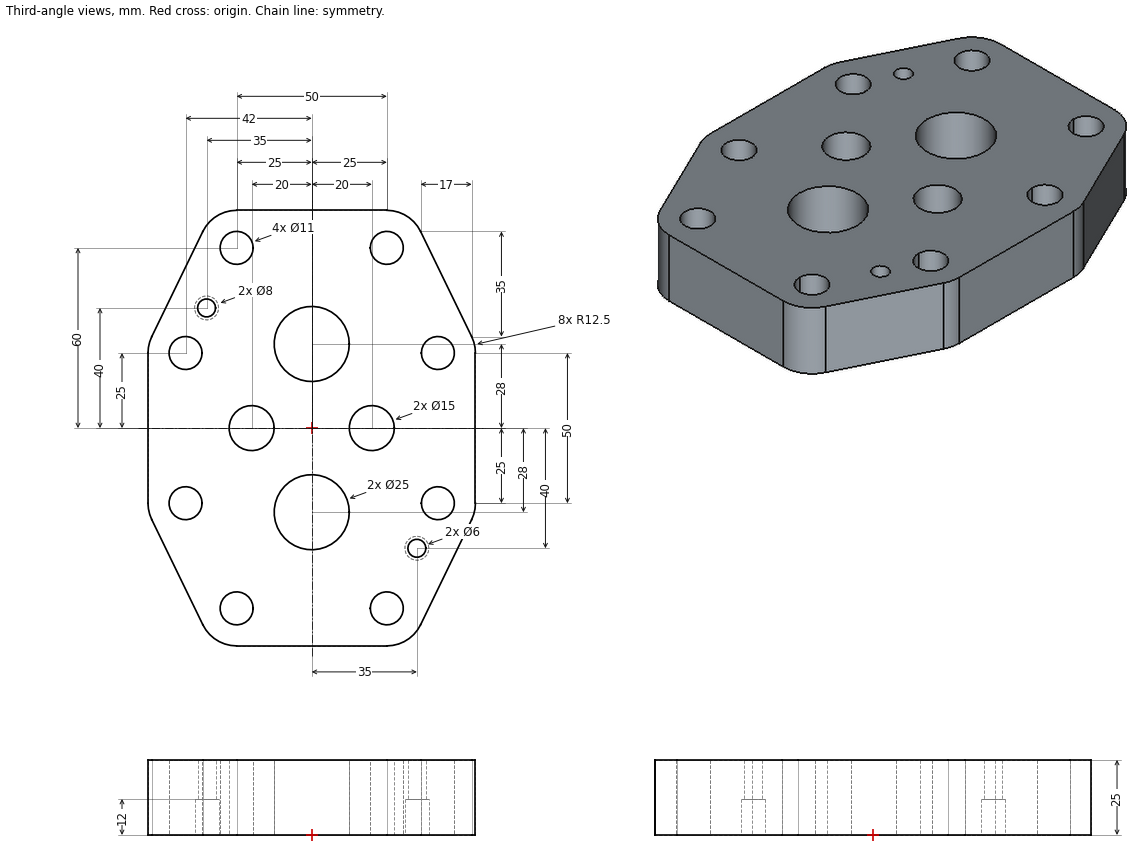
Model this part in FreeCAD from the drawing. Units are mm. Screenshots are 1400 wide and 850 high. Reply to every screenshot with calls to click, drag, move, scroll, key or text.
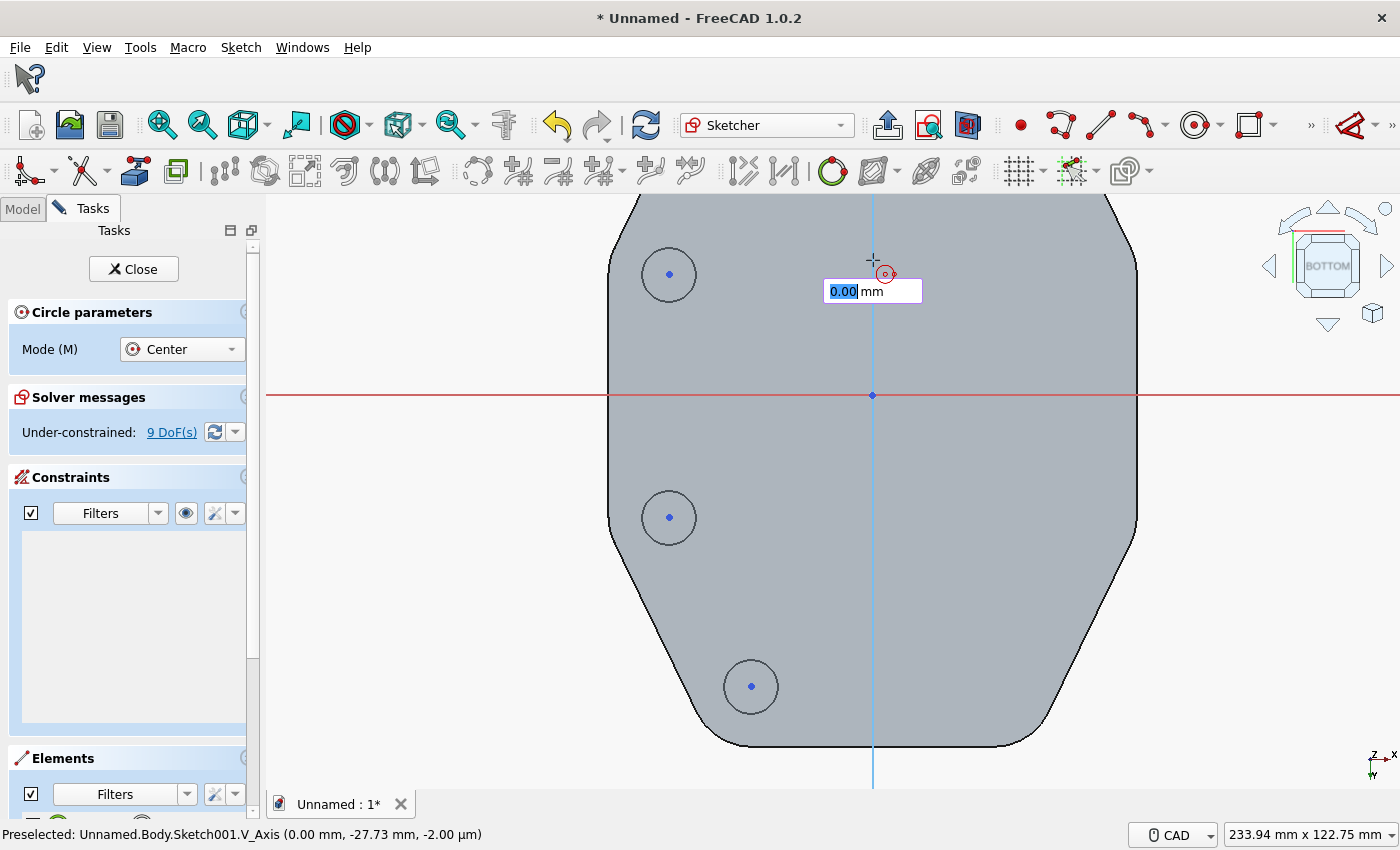
scroll(692, 608, down, 3)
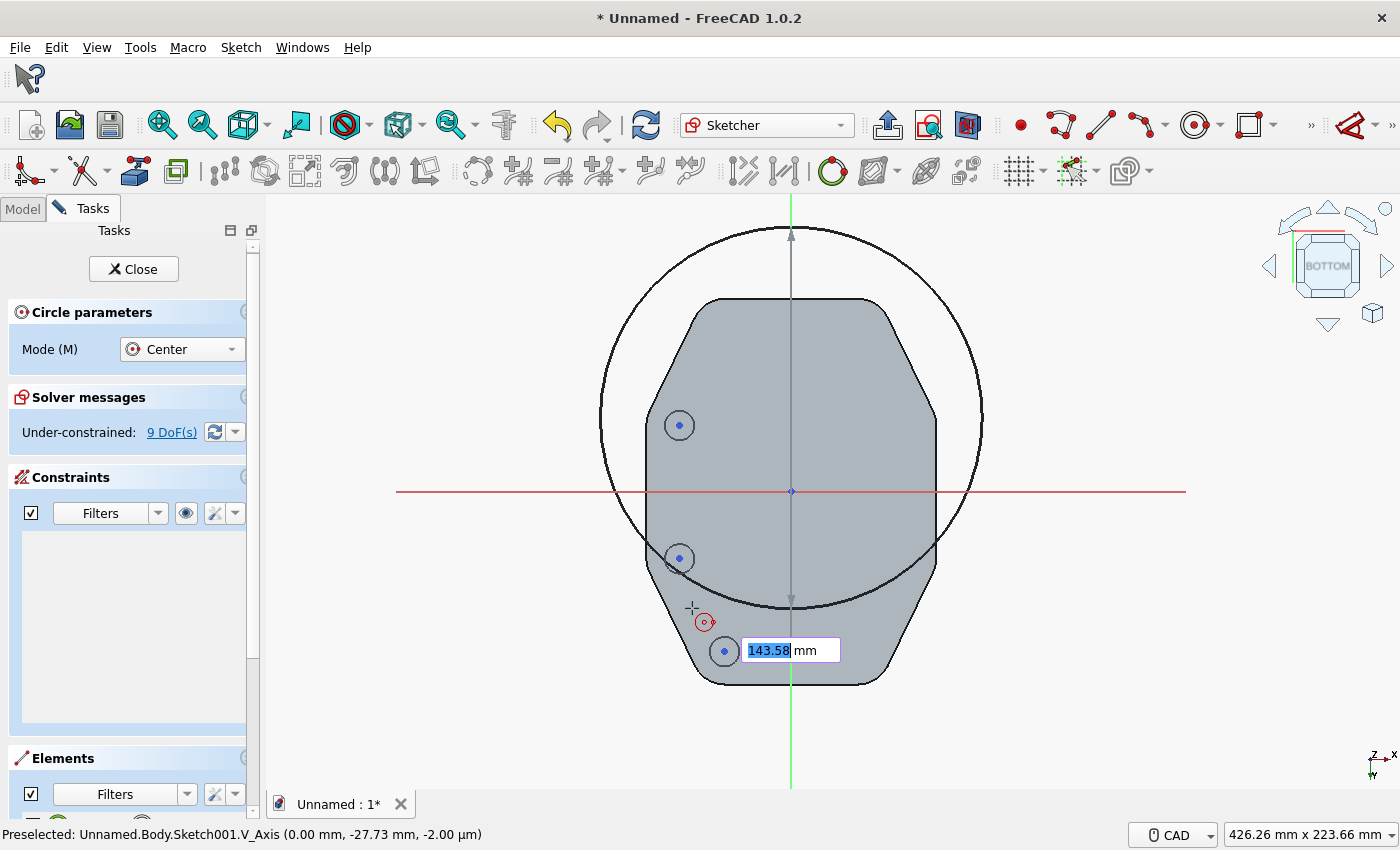
click(815, 394)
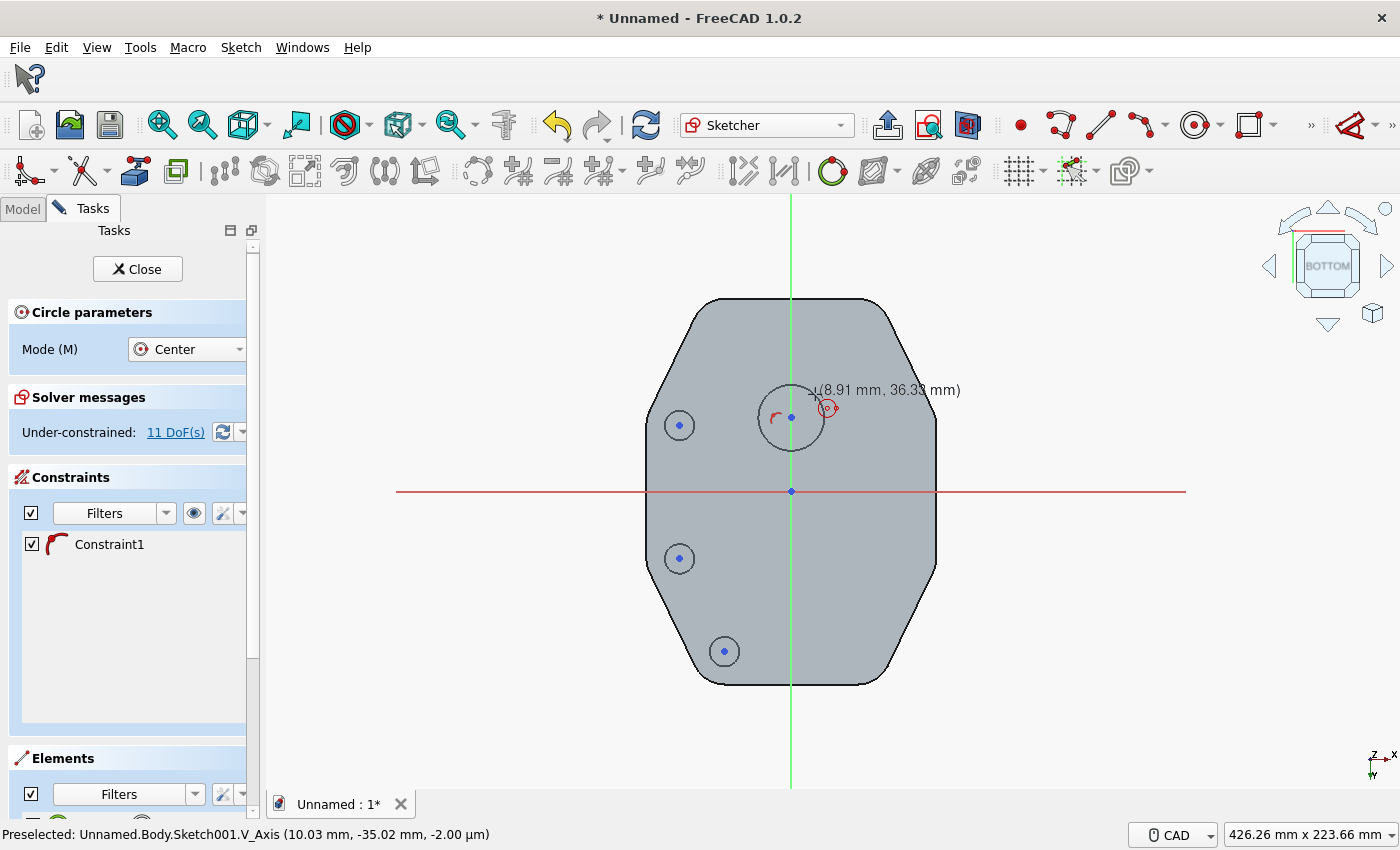
click(845, 492)
click(859, 478)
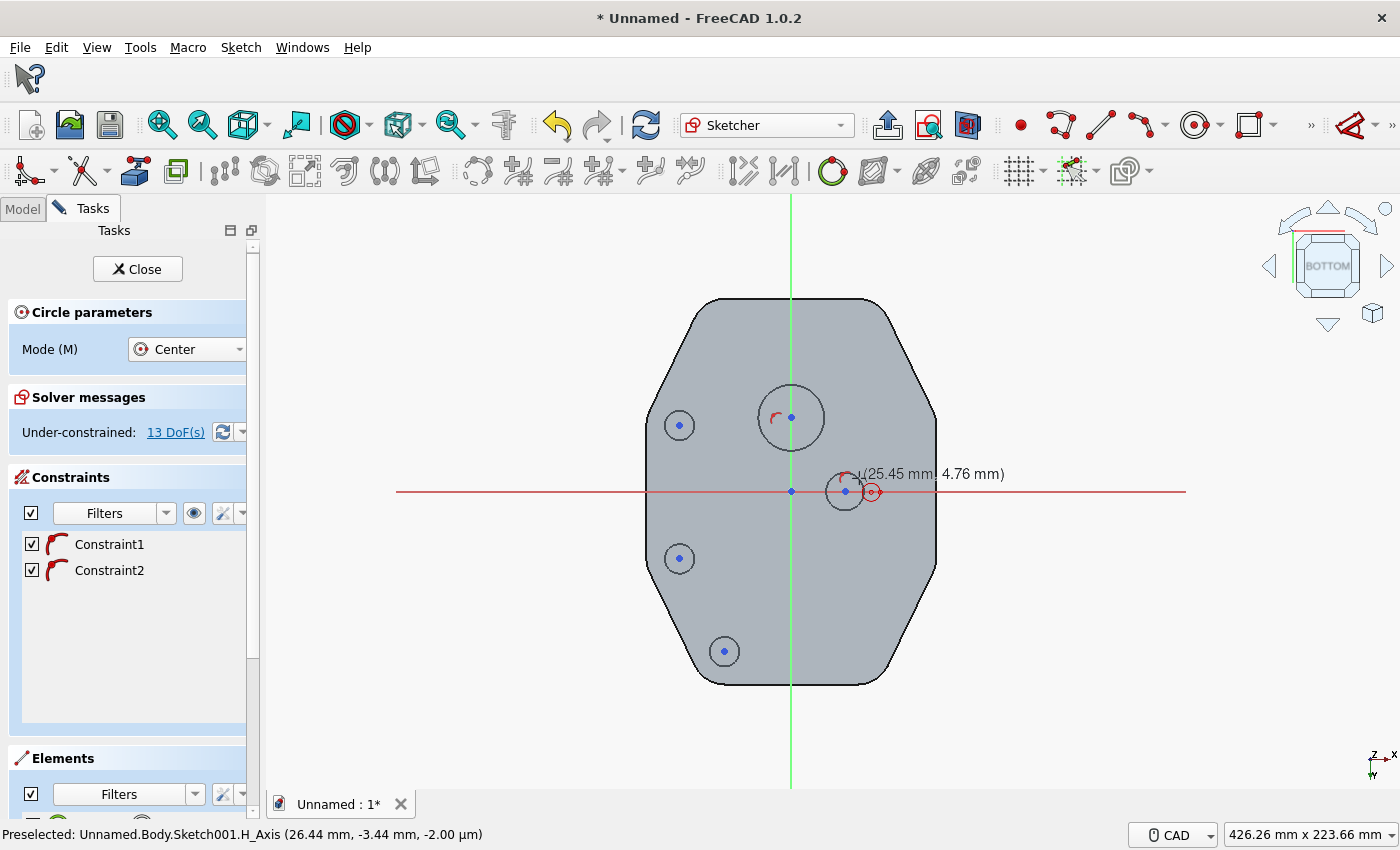
click(738, 492)
click(752, 478)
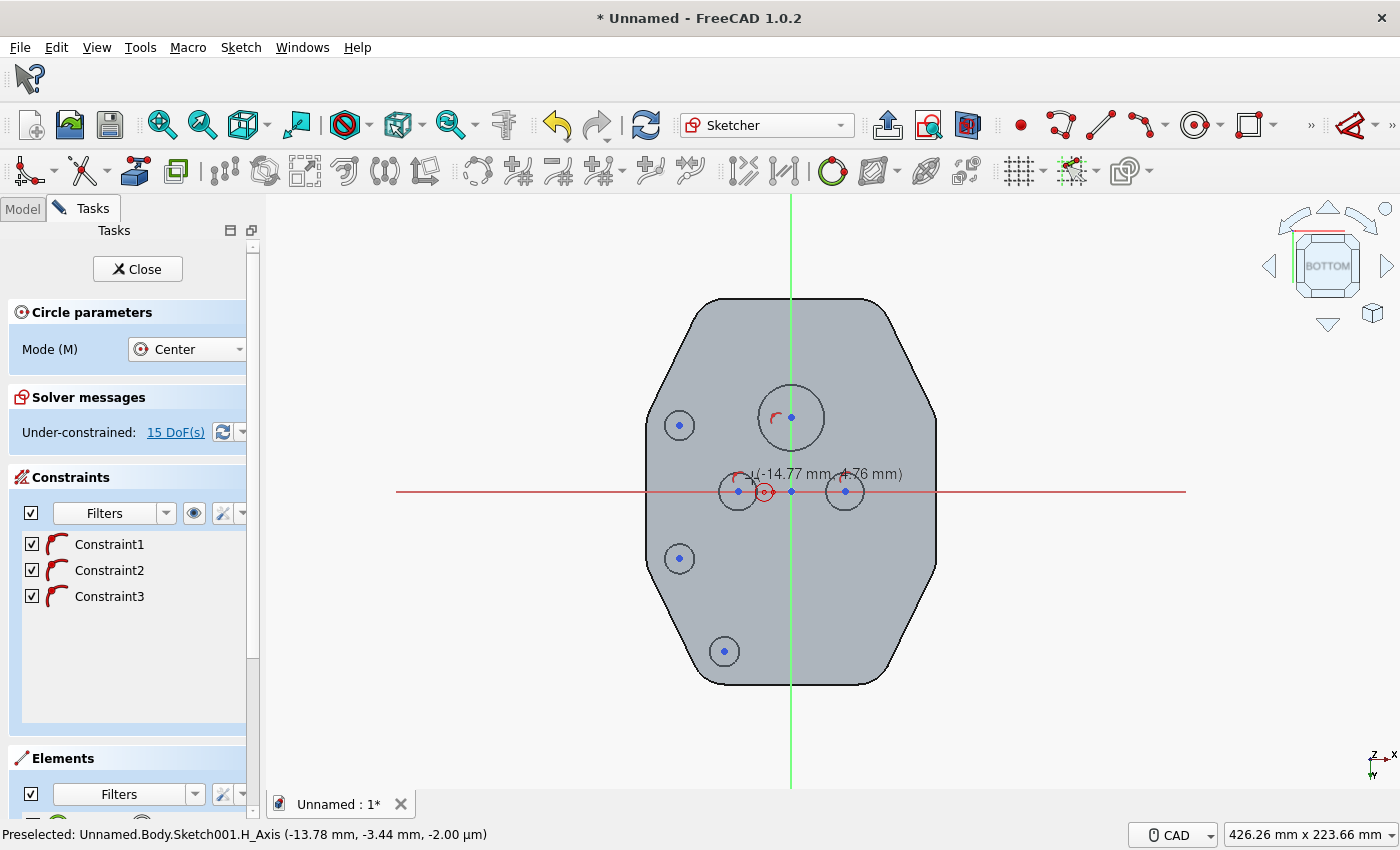
click(791, 566)
click(815, 543)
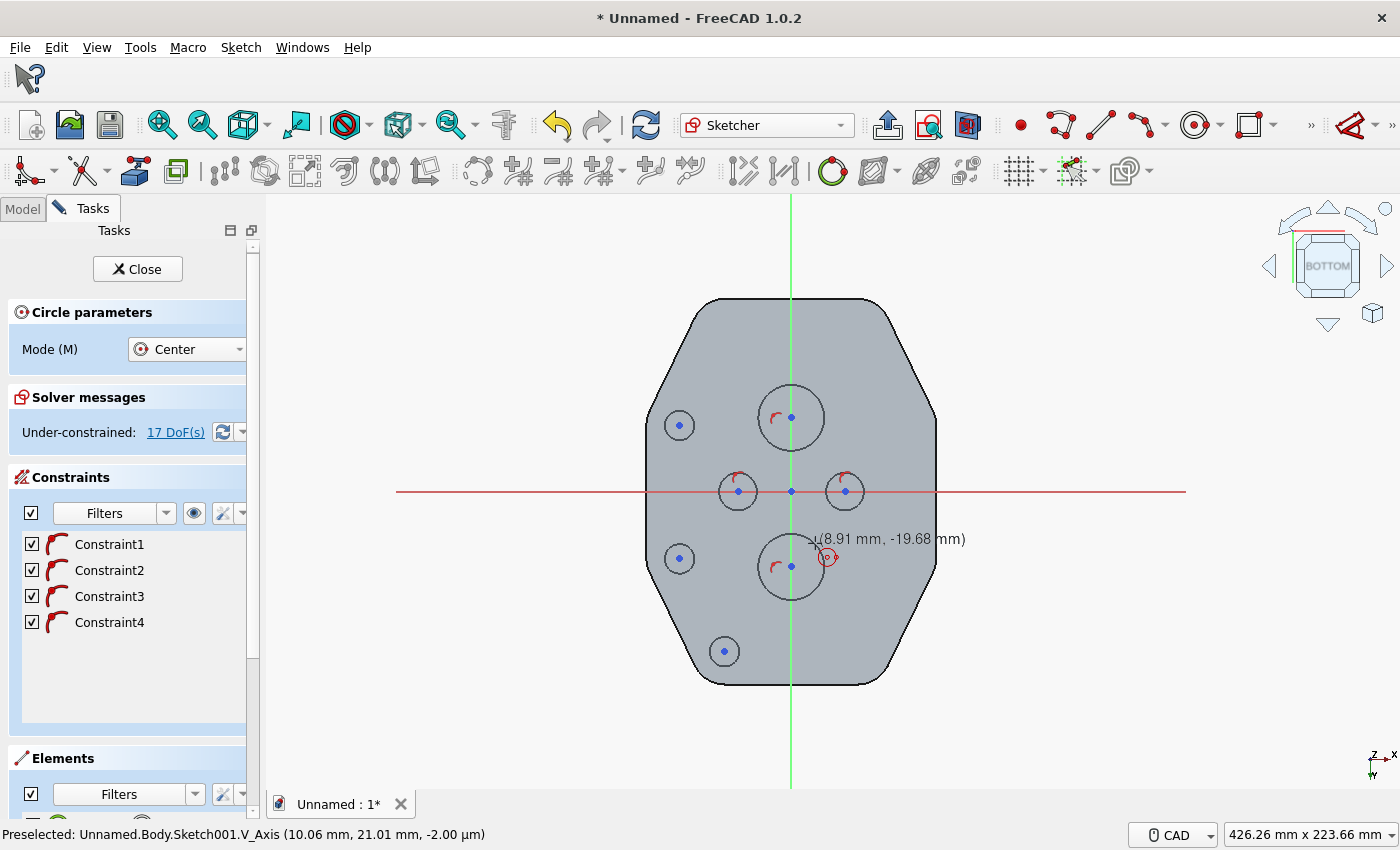
scroll(725, 332, up, 3)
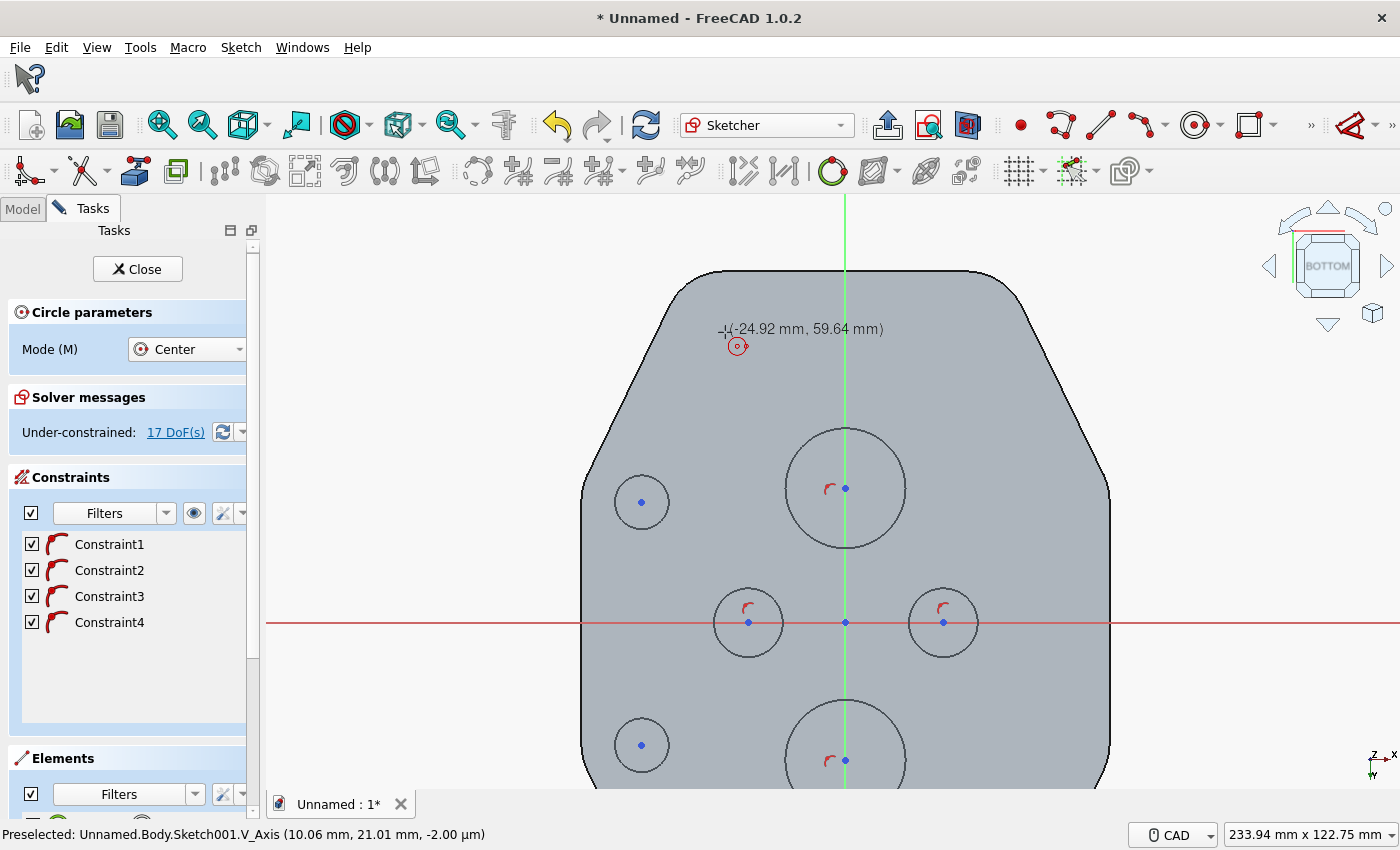
click(724, 332)
click(743, 313)
key(Escape)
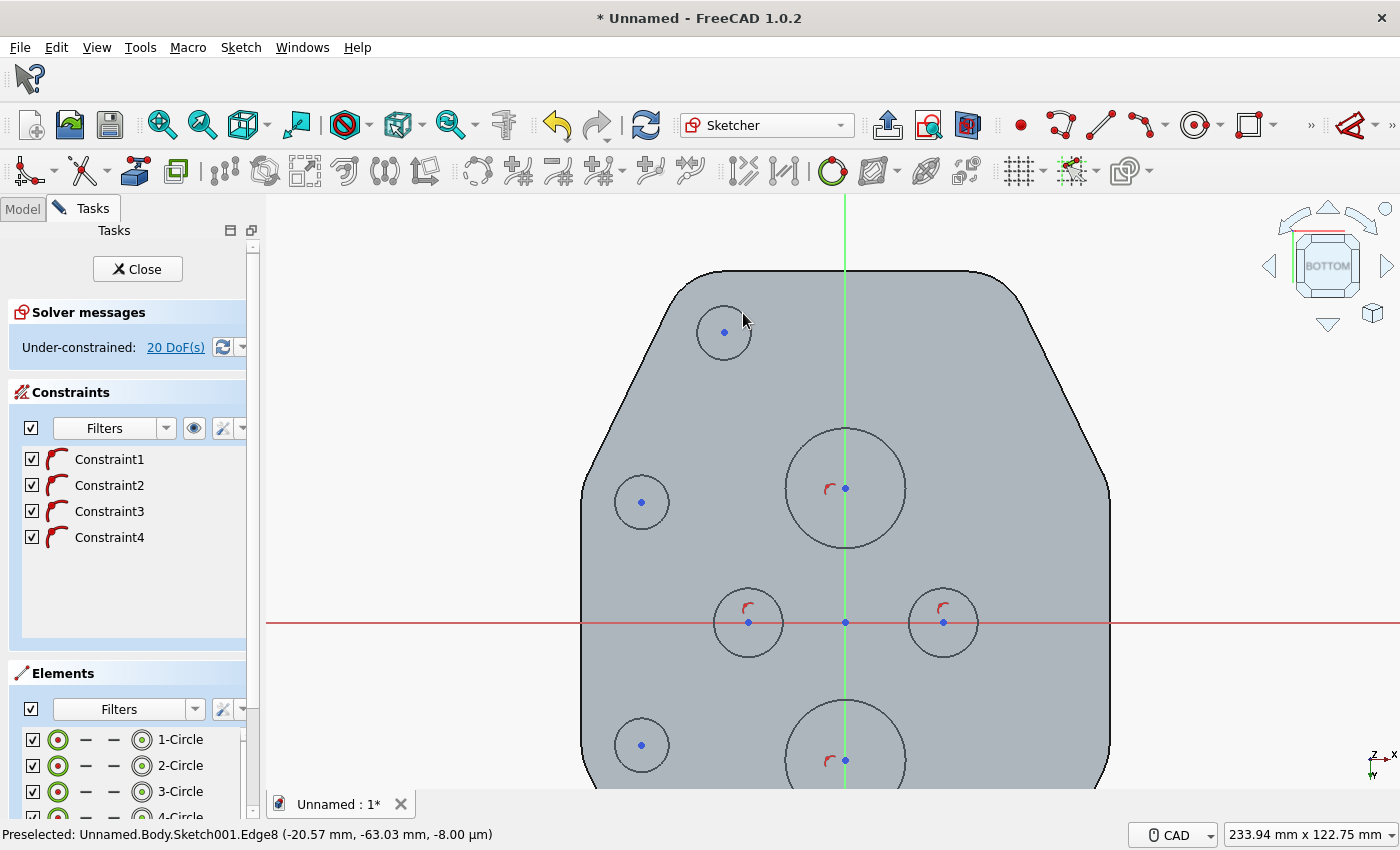
scroll(725, 332, down, 3)